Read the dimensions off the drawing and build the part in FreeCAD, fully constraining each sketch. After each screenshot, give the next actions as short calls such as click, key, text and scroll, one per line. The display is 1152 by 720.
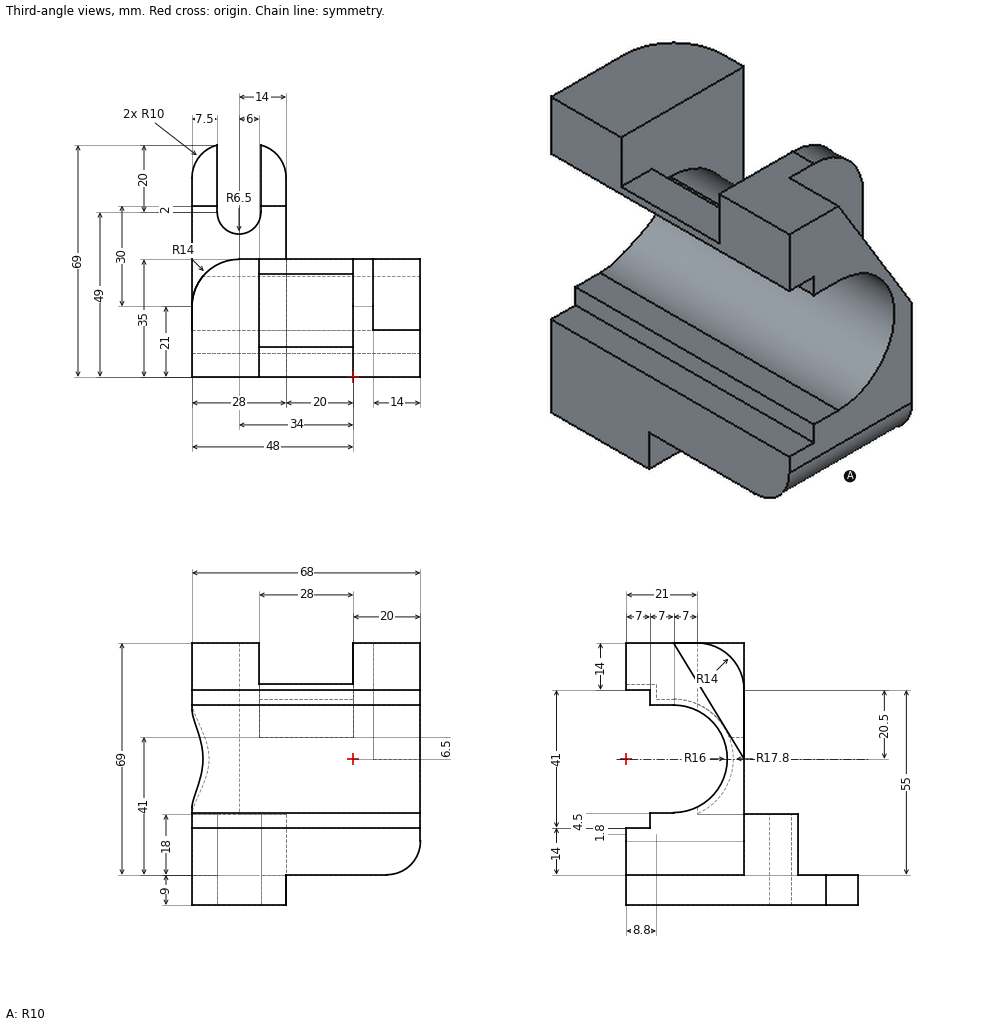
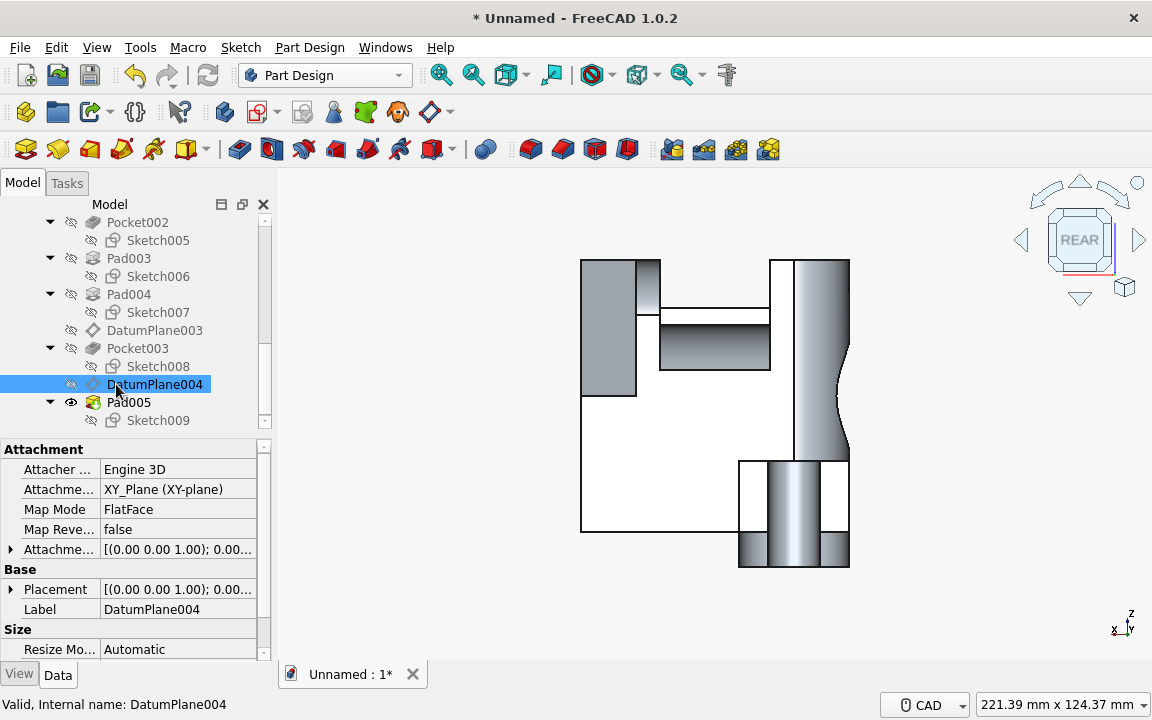
key(0)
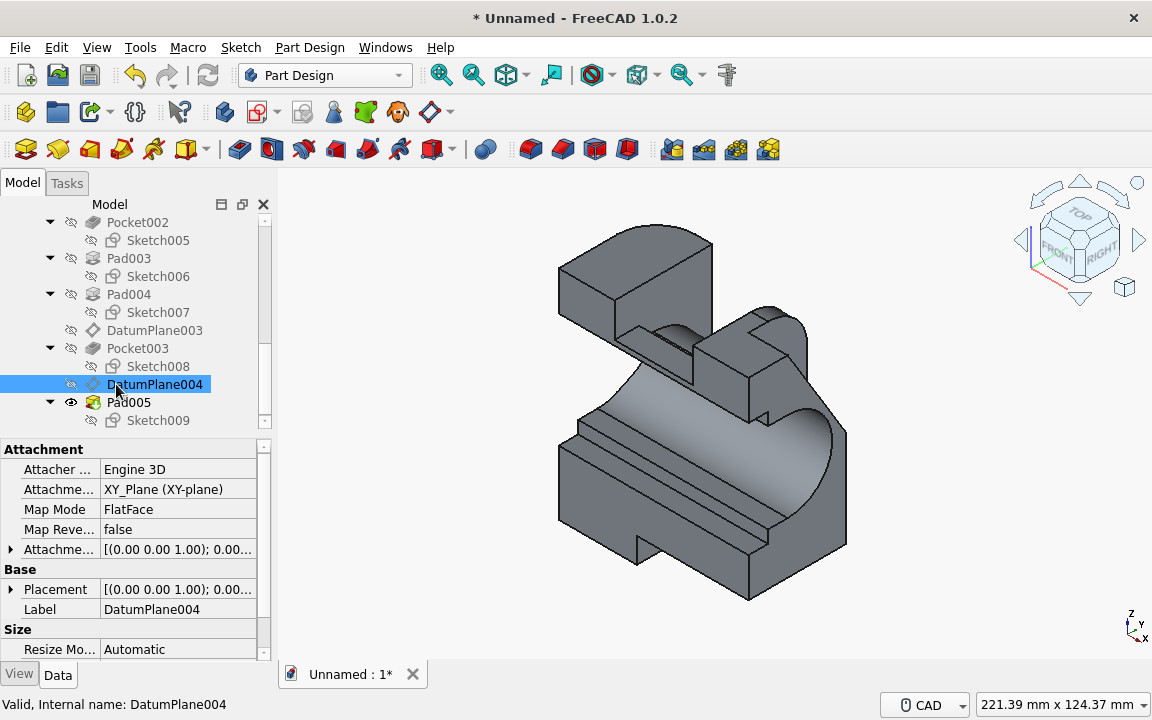
click(442, 76)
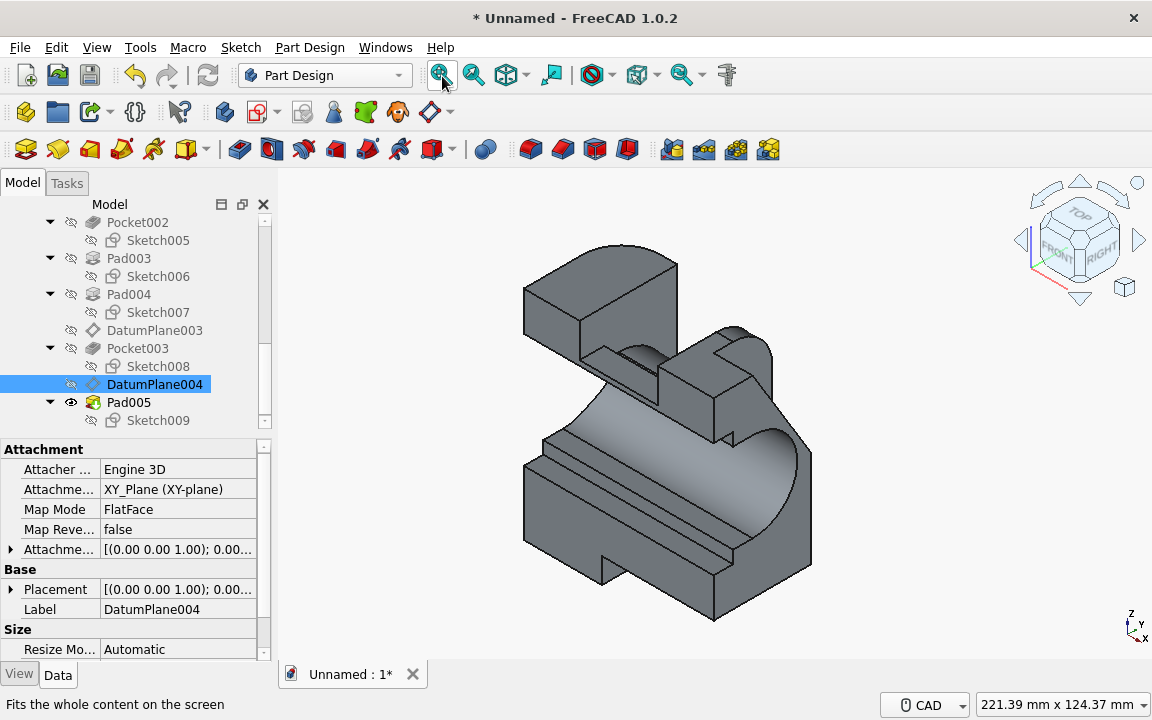
key(2)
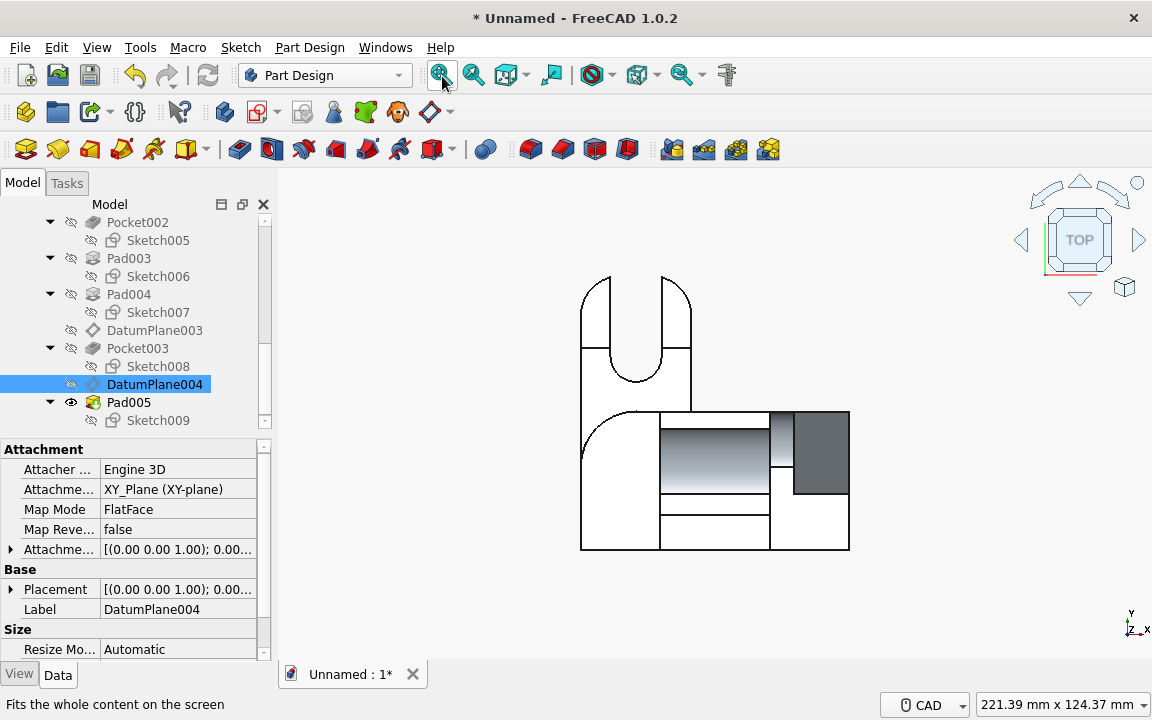
key(1)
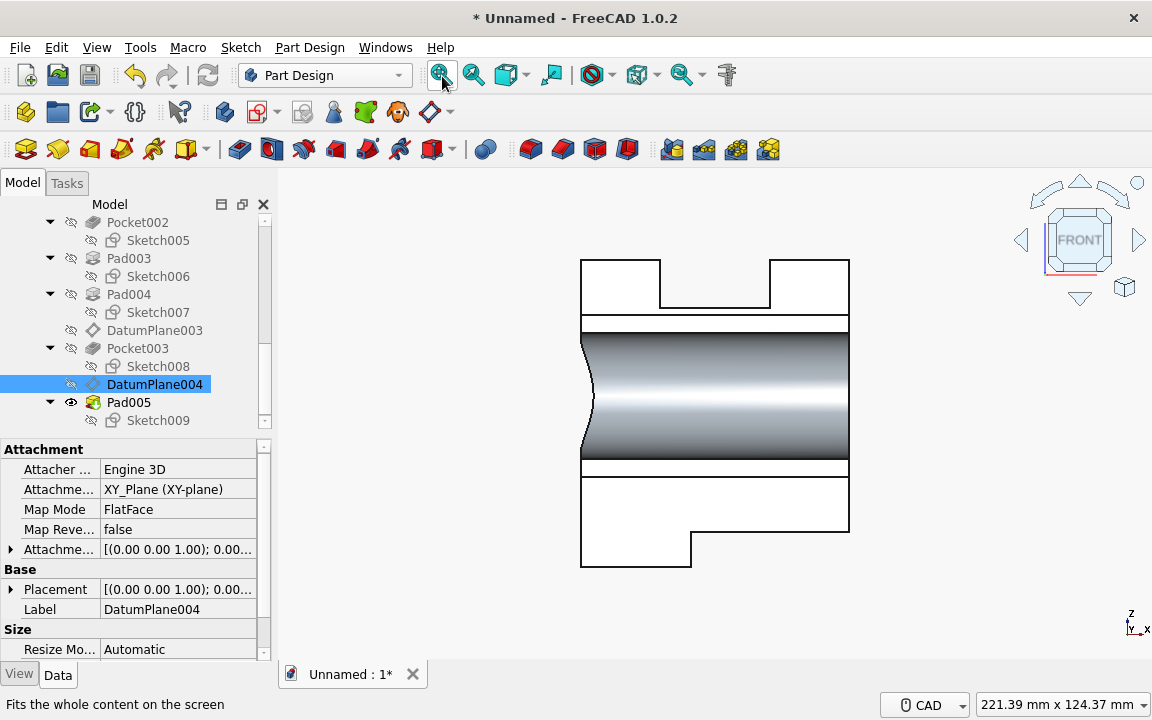
key(3)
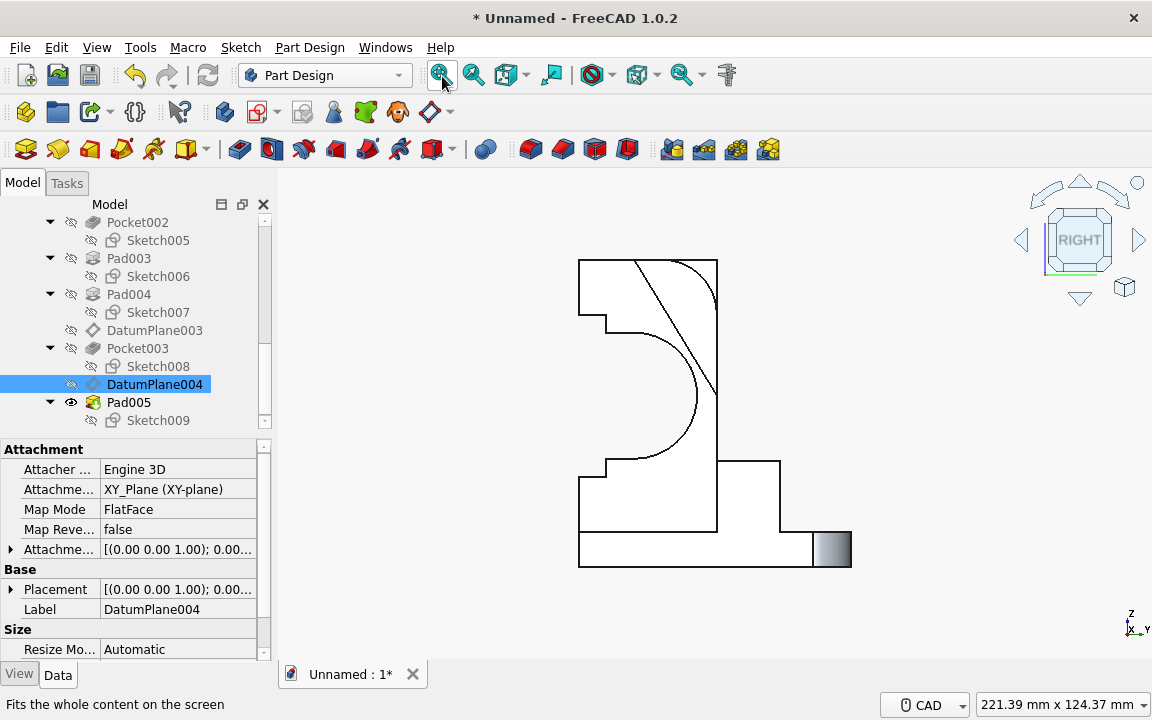
click(648, 531)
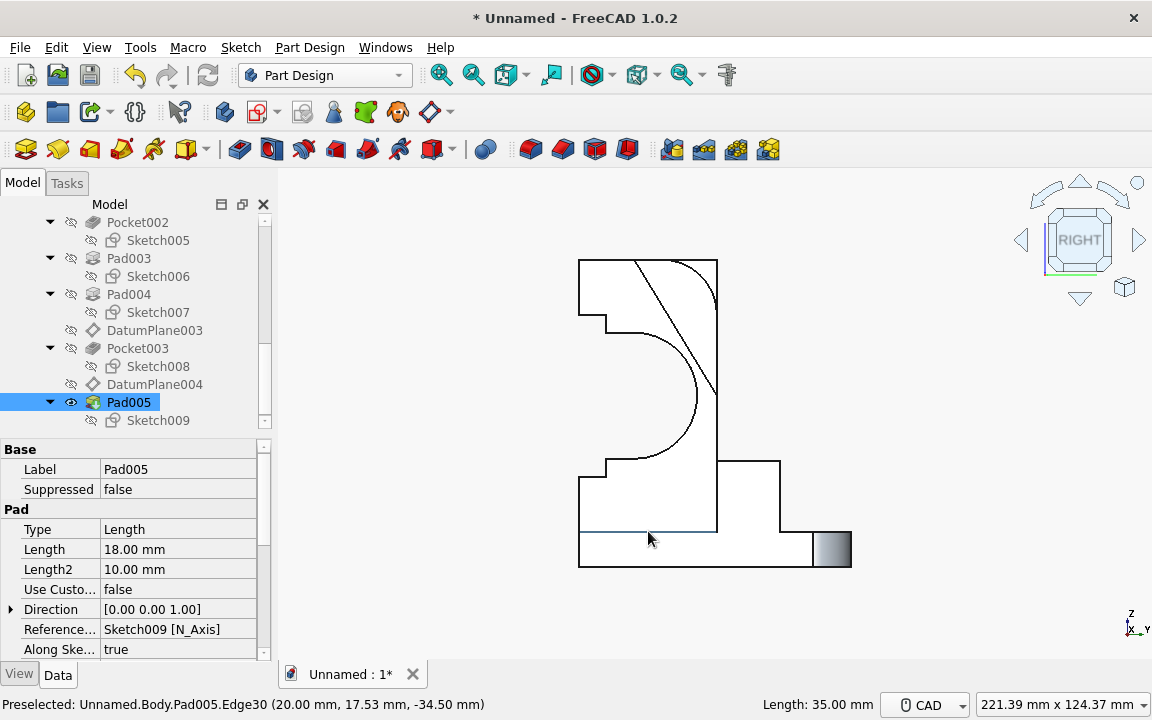
click(532, 150)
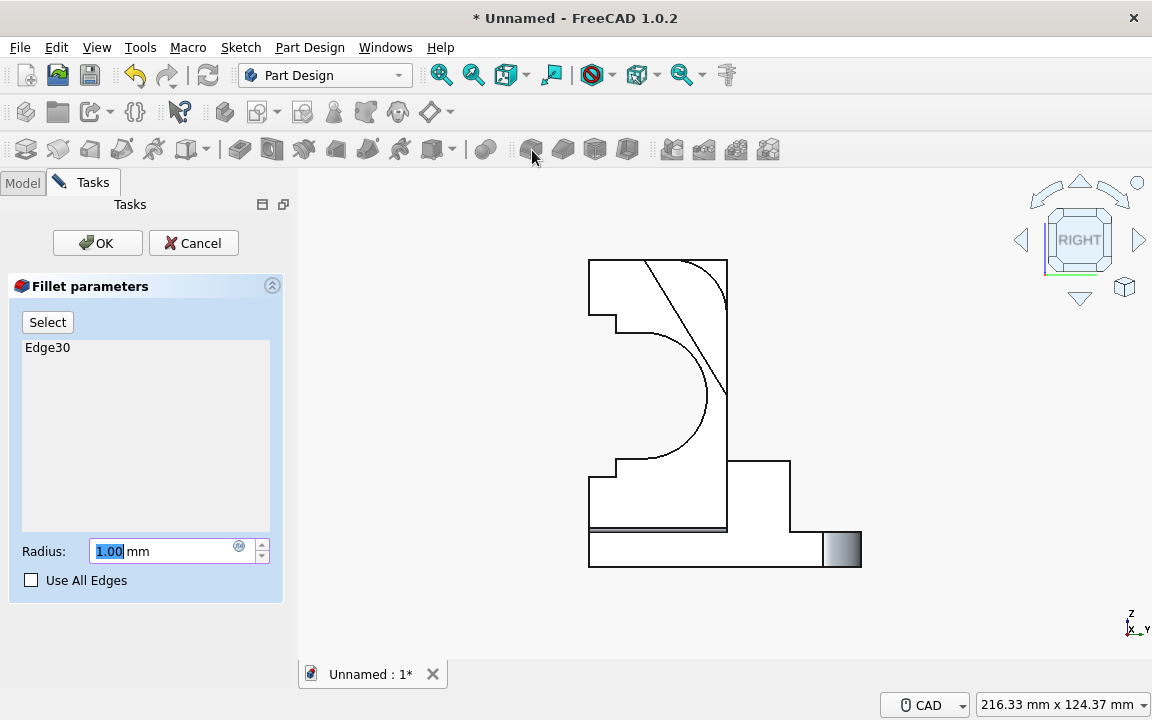
text(10)
key(Tab)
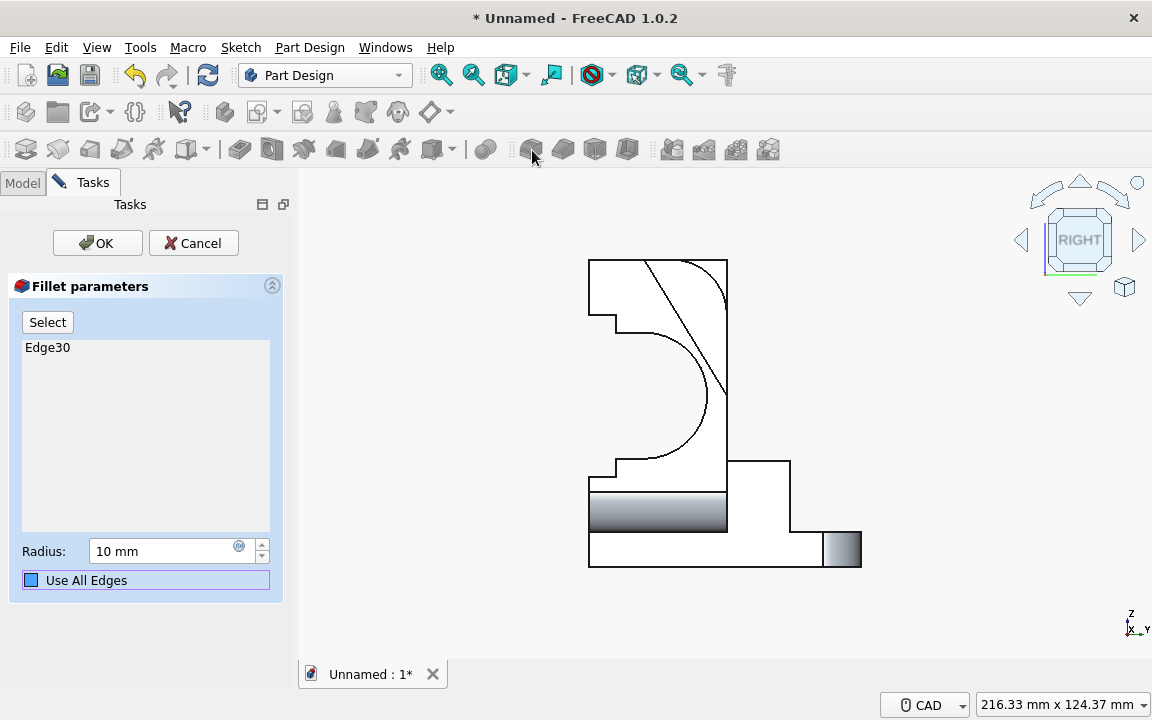
click(98, 243)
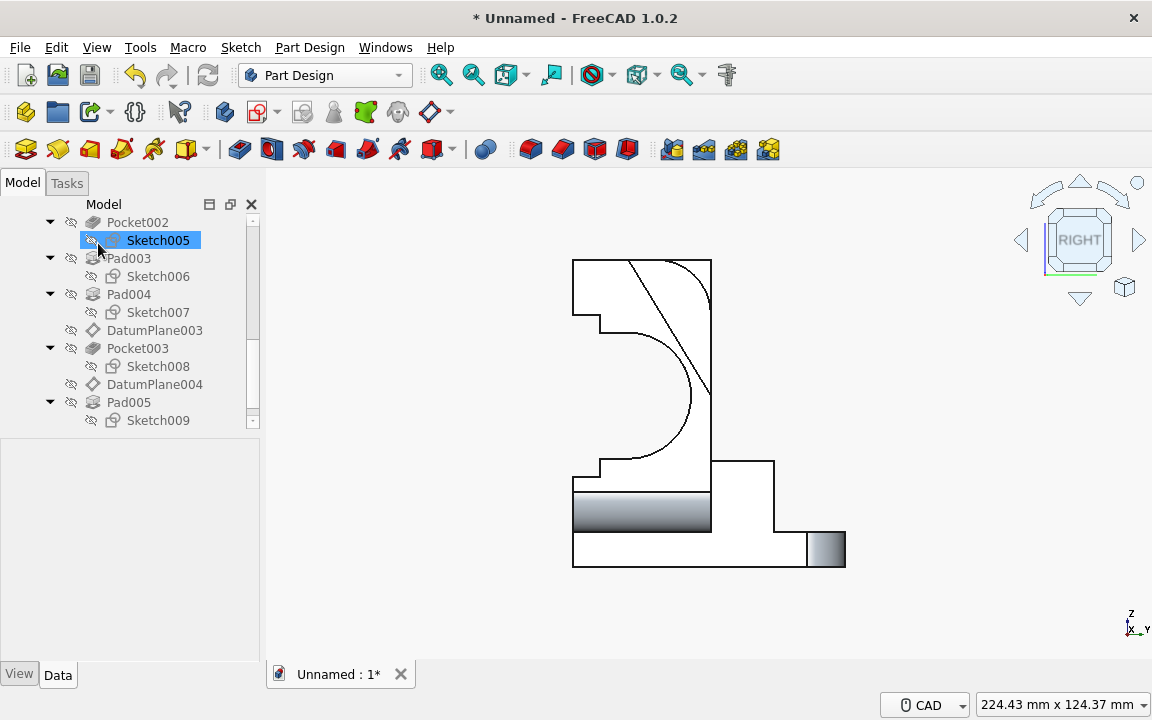
key(0)